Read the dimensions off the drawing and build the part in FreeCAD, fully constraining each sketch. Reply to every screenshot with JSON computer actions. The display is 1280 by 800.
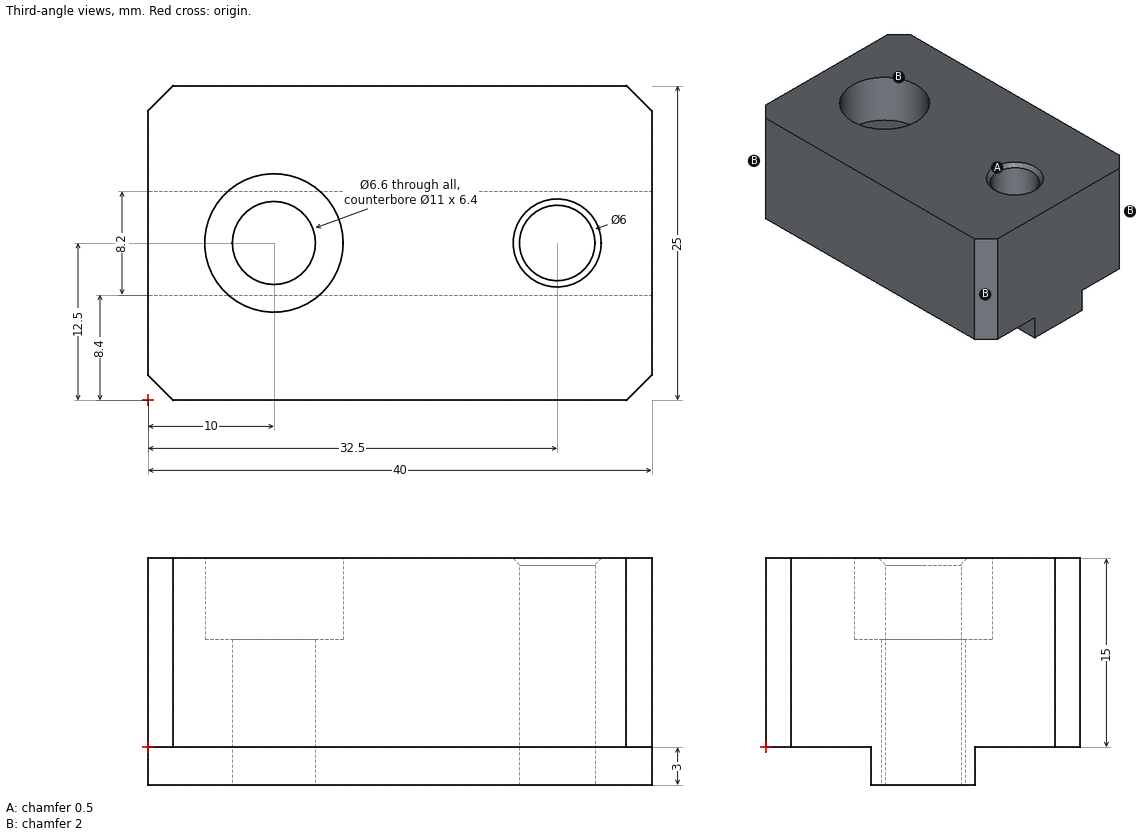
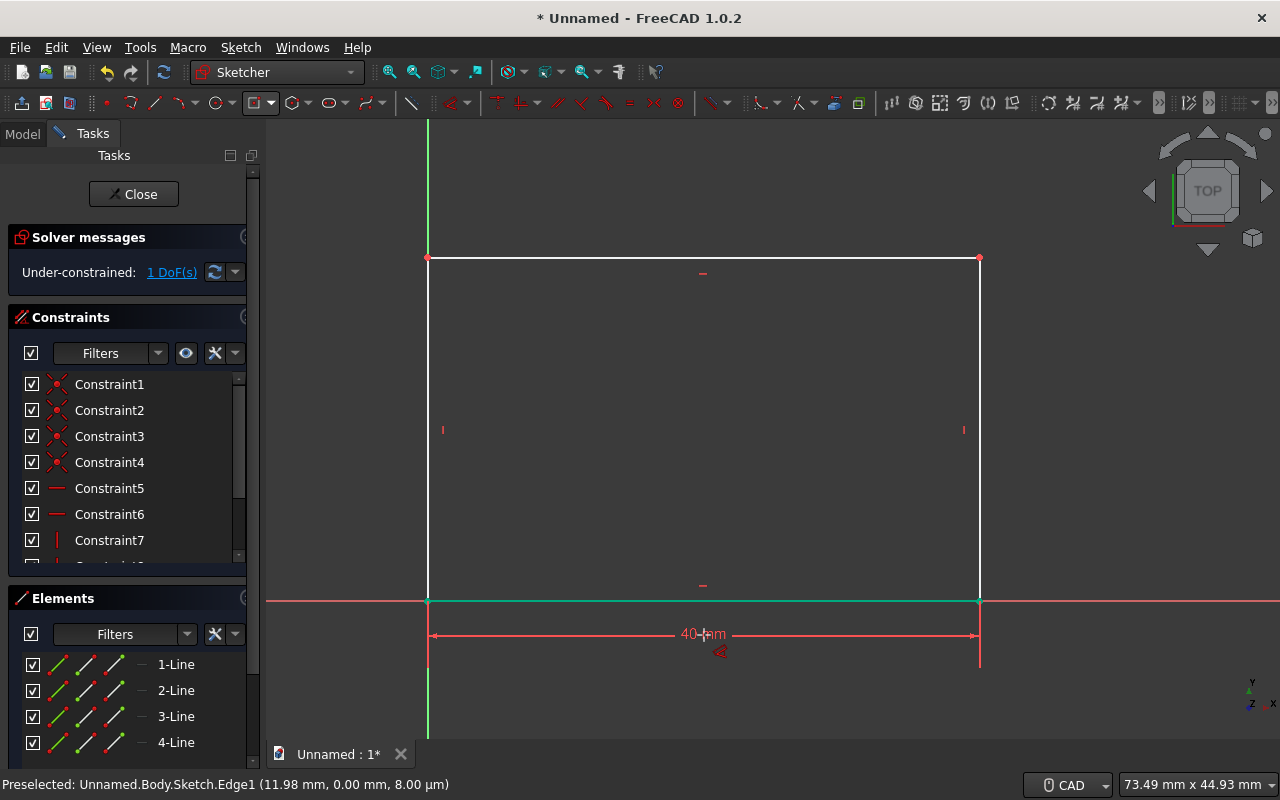
{"action": "left_click", "coordinate": [980, 498]}
{"action": "left_click", "coordinate": [1014, 430]}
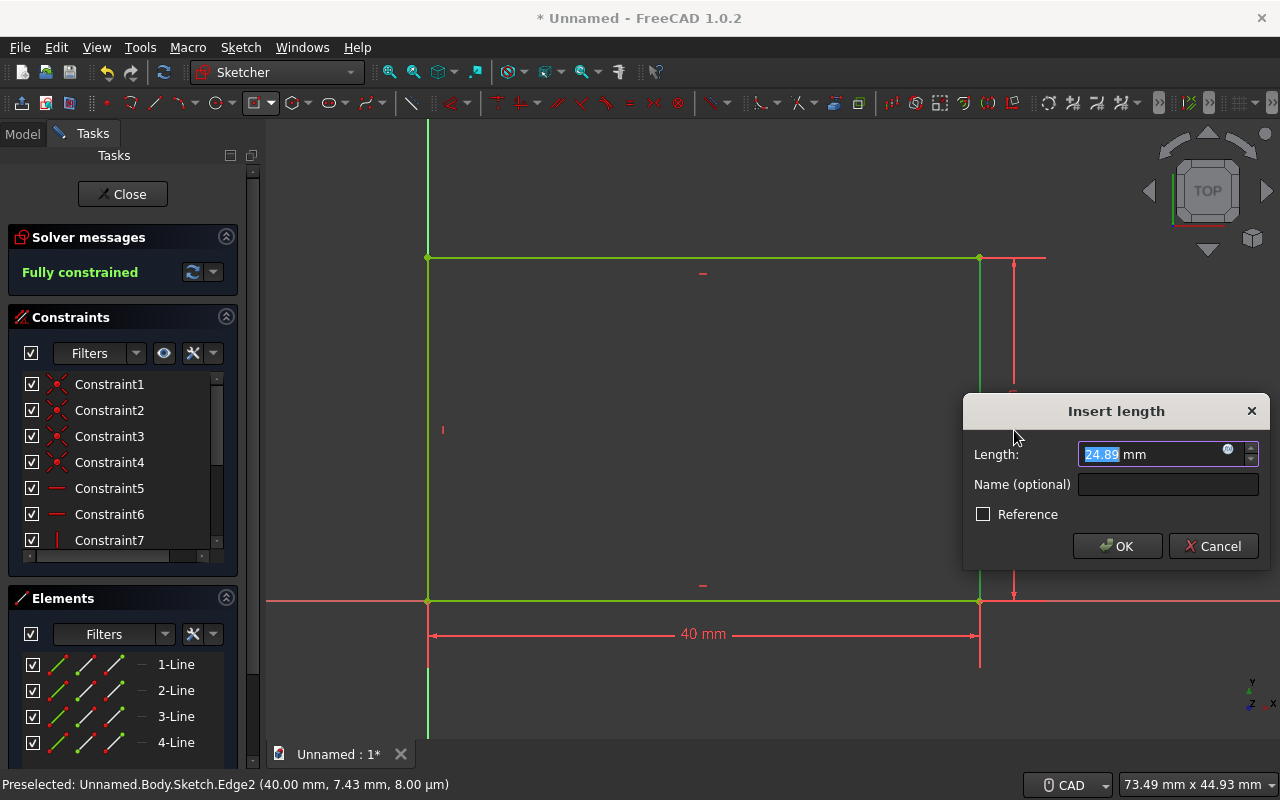
{"action": "type", "text": "25"}
{"action": "key", "text": "Return"}
{"action": "key", "text": "Escape"}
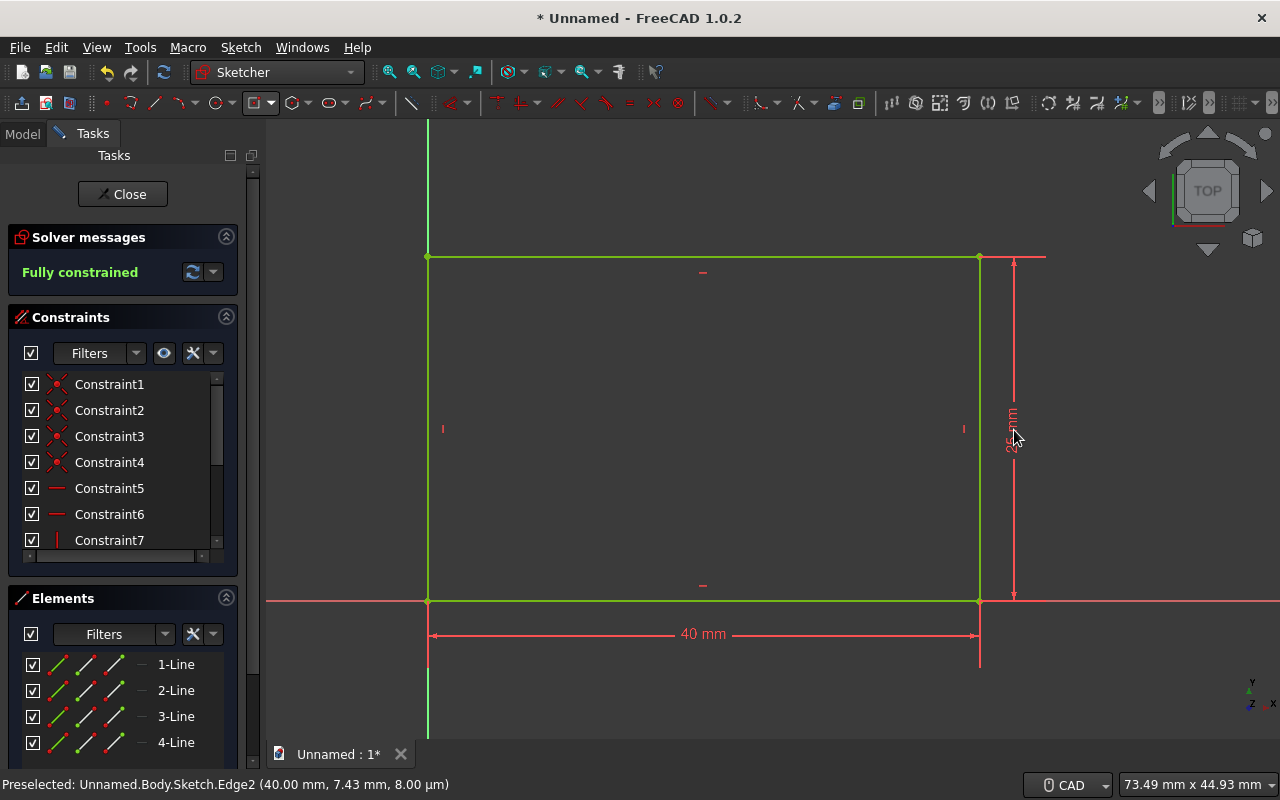
{"action": "left_click", "coordinate": [123, 194]}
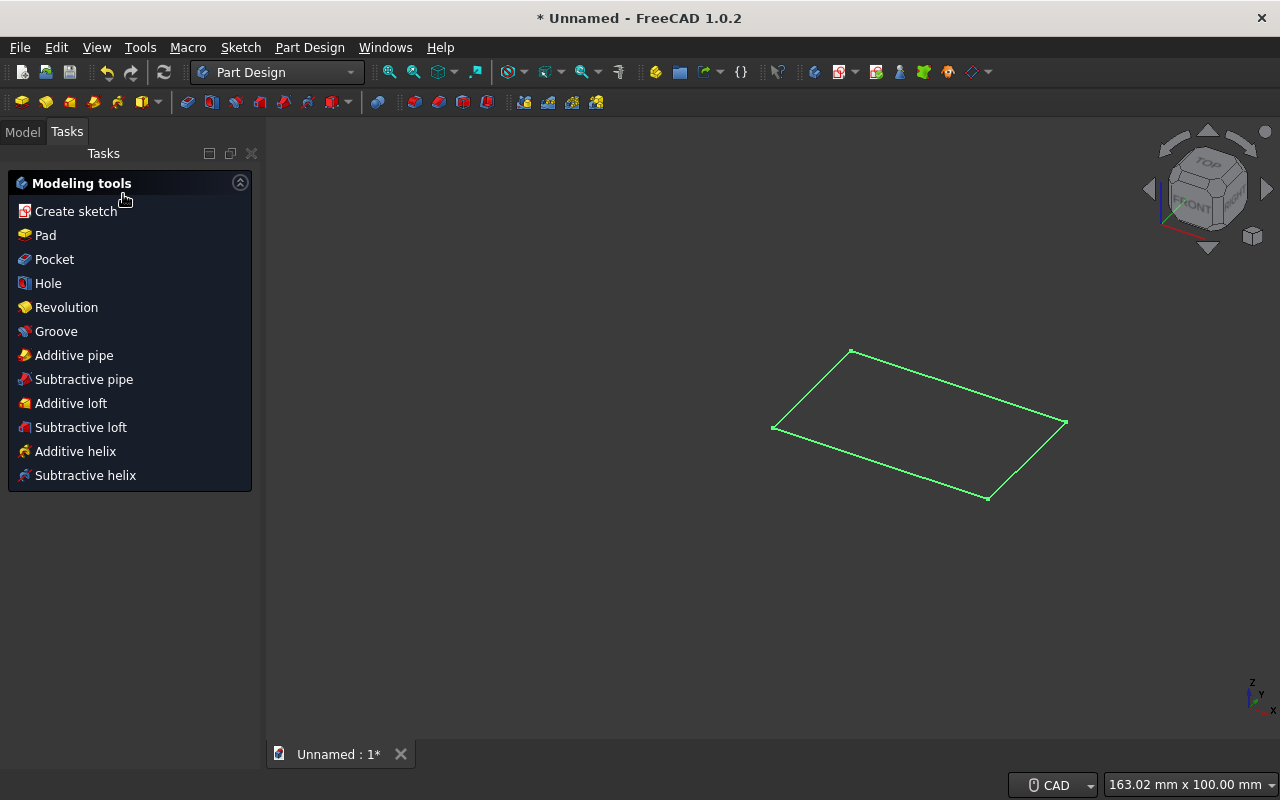
{"action": "left_click", "coordinate": [22, 102]}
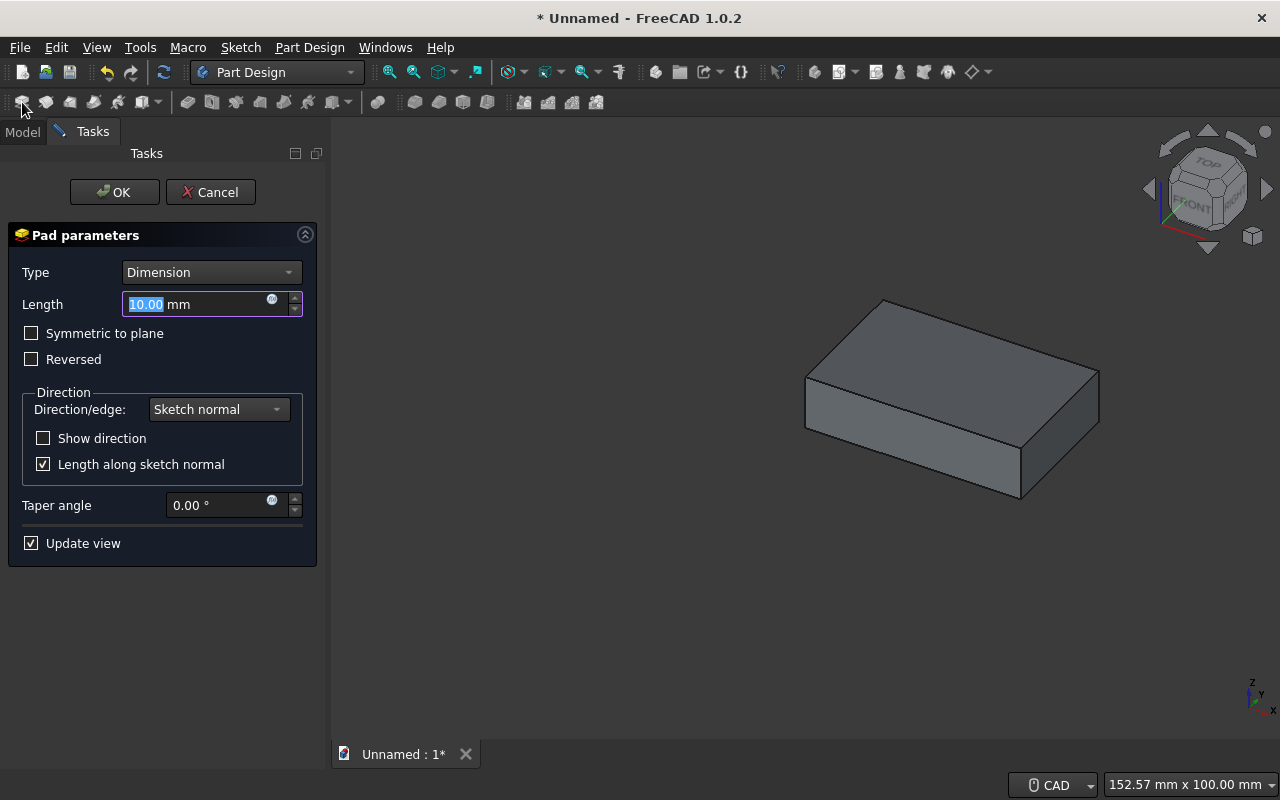
{"action": "type", "text": "15"}
{"action": "key", "text": "Tab"}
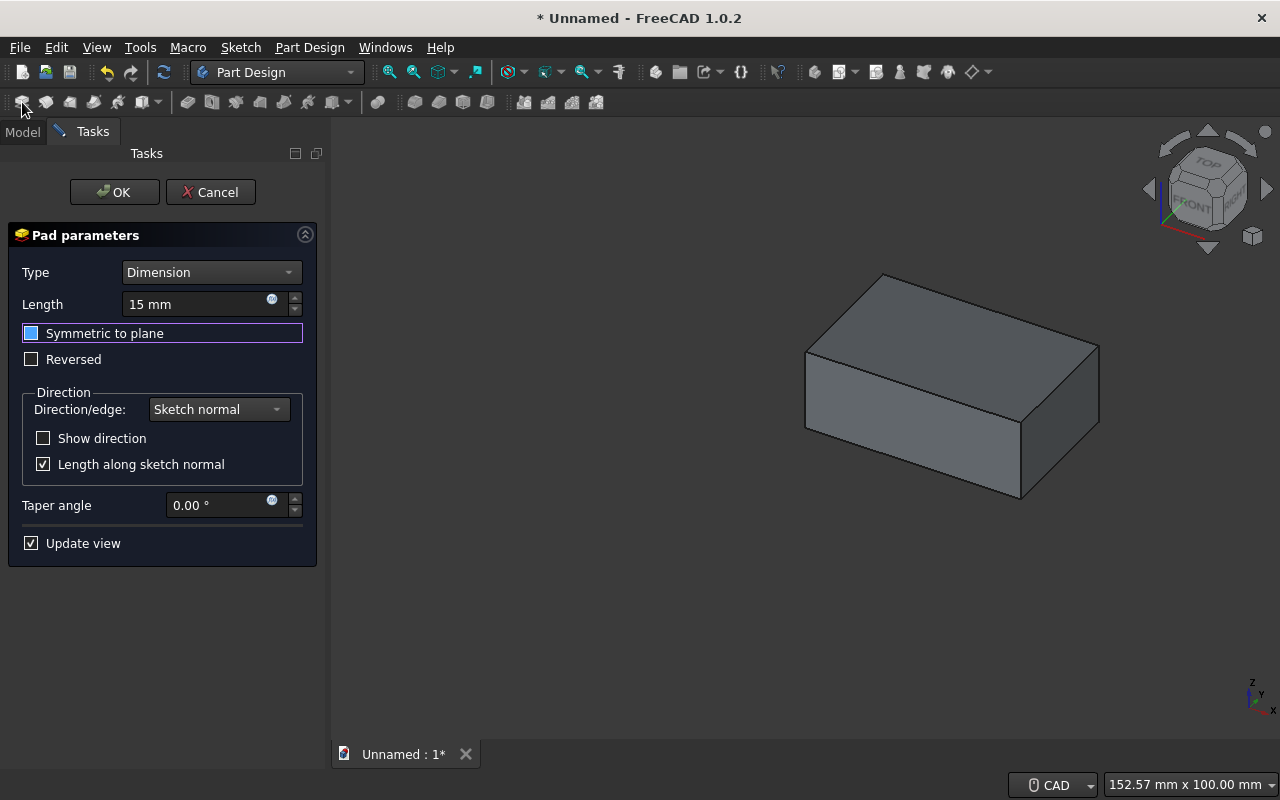
{"action": "left_click", "coordinate": [115, 192]}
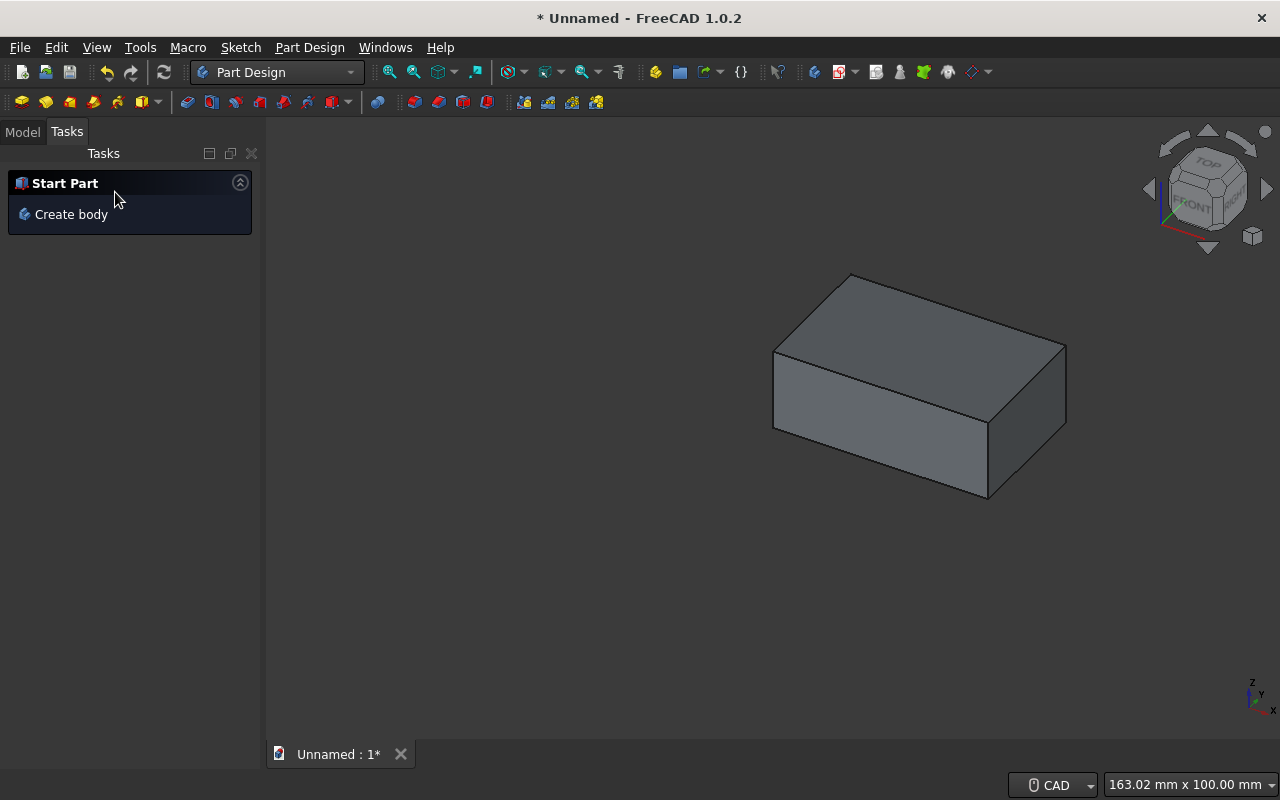
{"action": "left_click", "coordinate": [390, 72]}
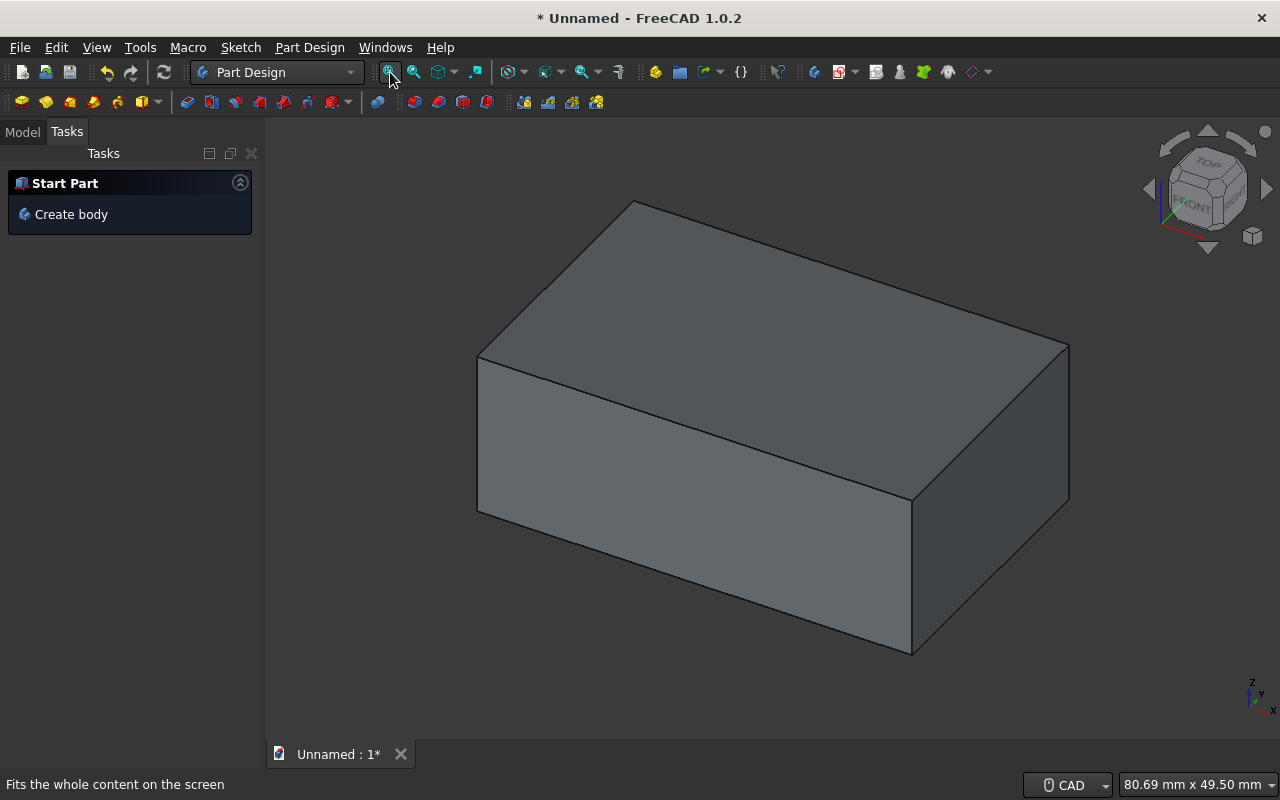
{"action": "key", "text": "5"}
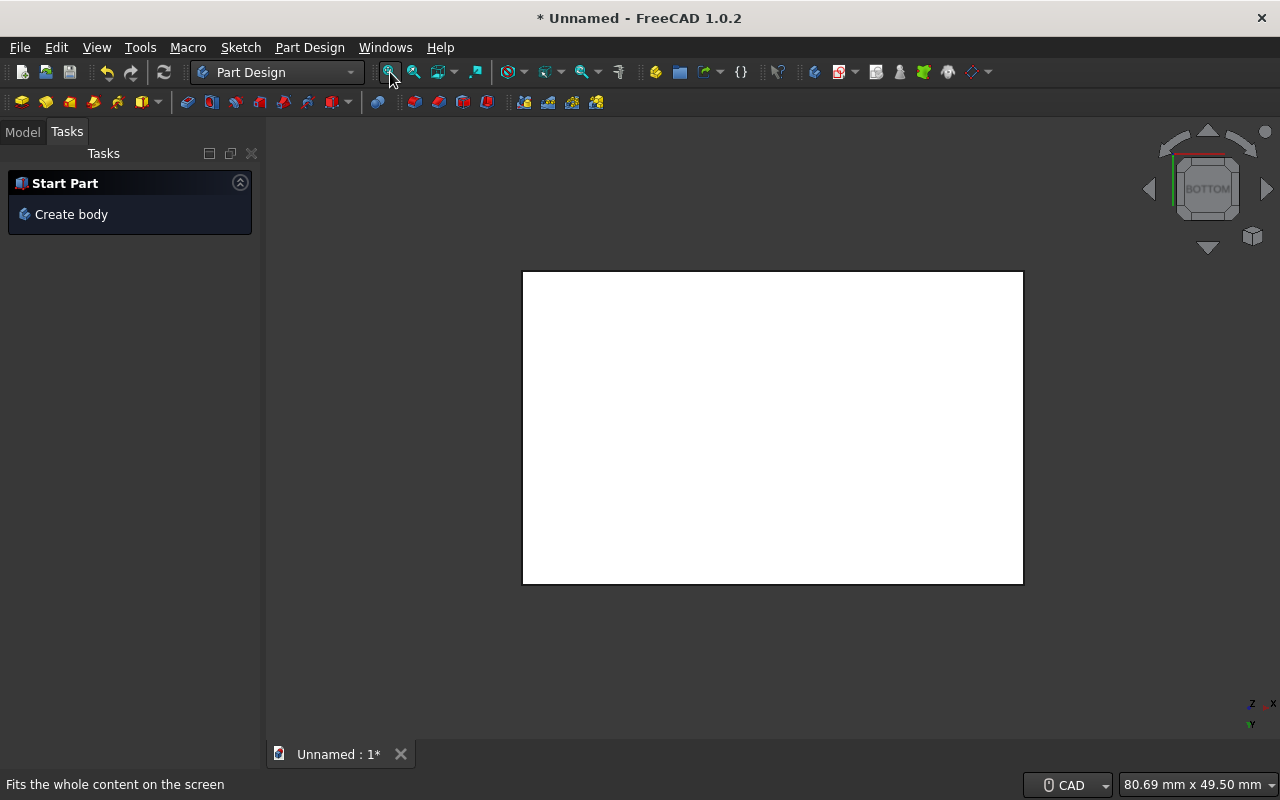
{"action": "left_click", "coordinate": [845, 427]}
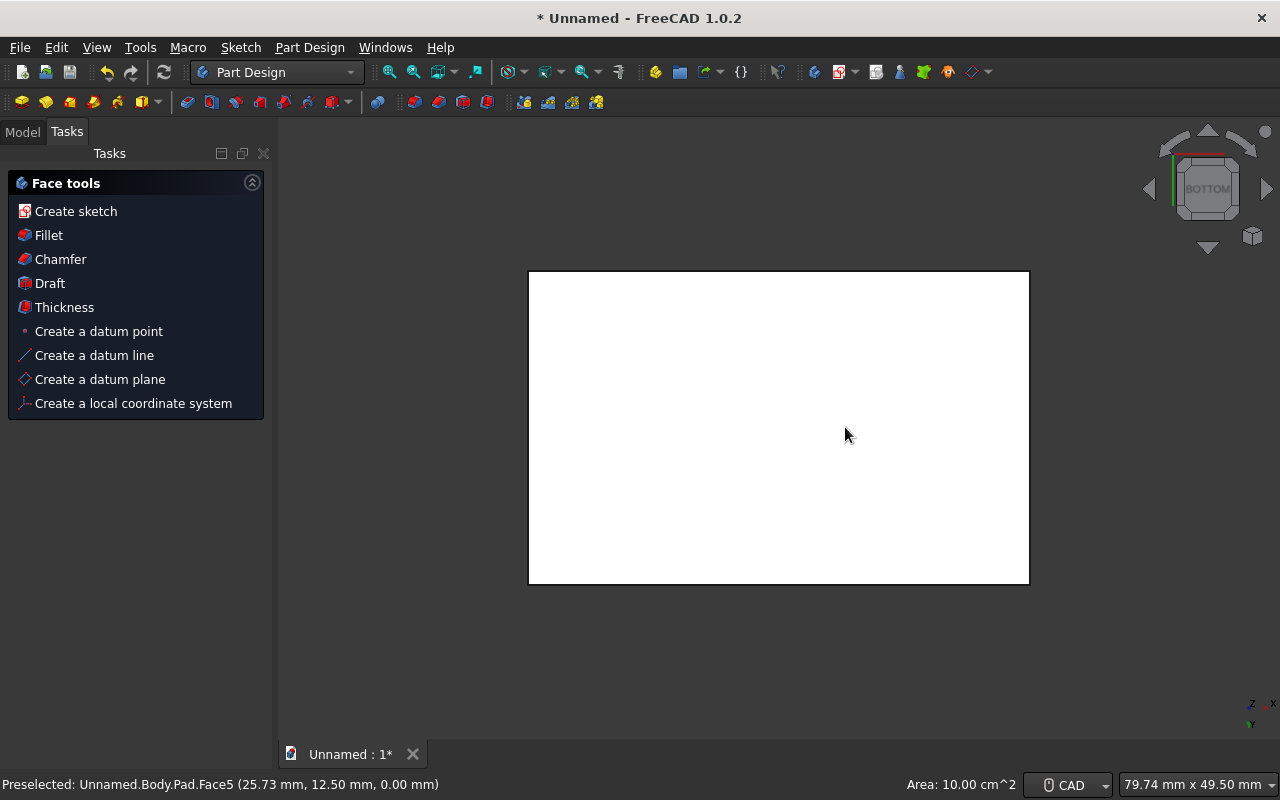
{"action": "left_click", "coordinate": [840, 72]}